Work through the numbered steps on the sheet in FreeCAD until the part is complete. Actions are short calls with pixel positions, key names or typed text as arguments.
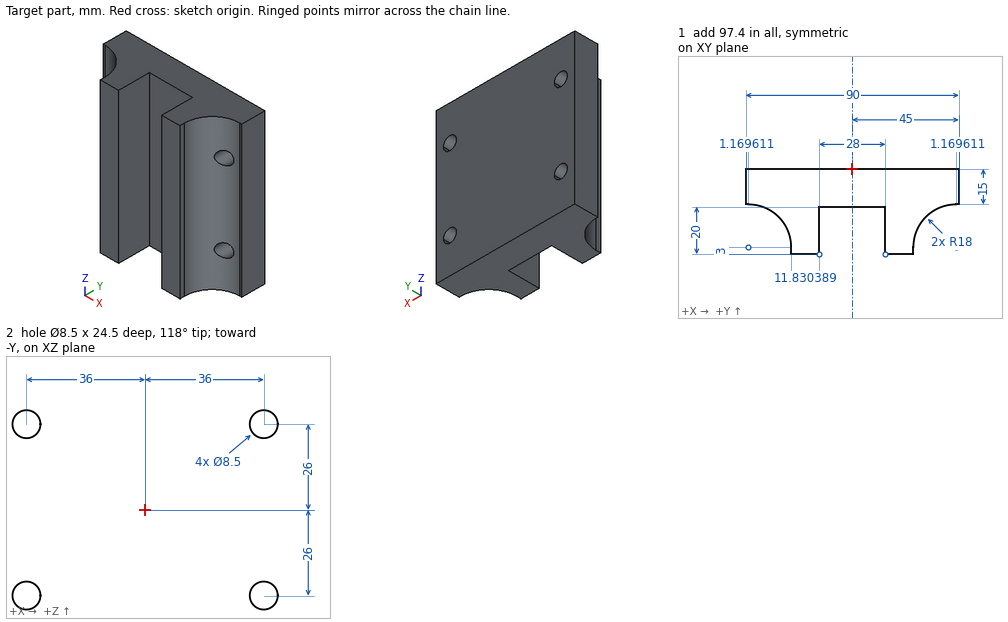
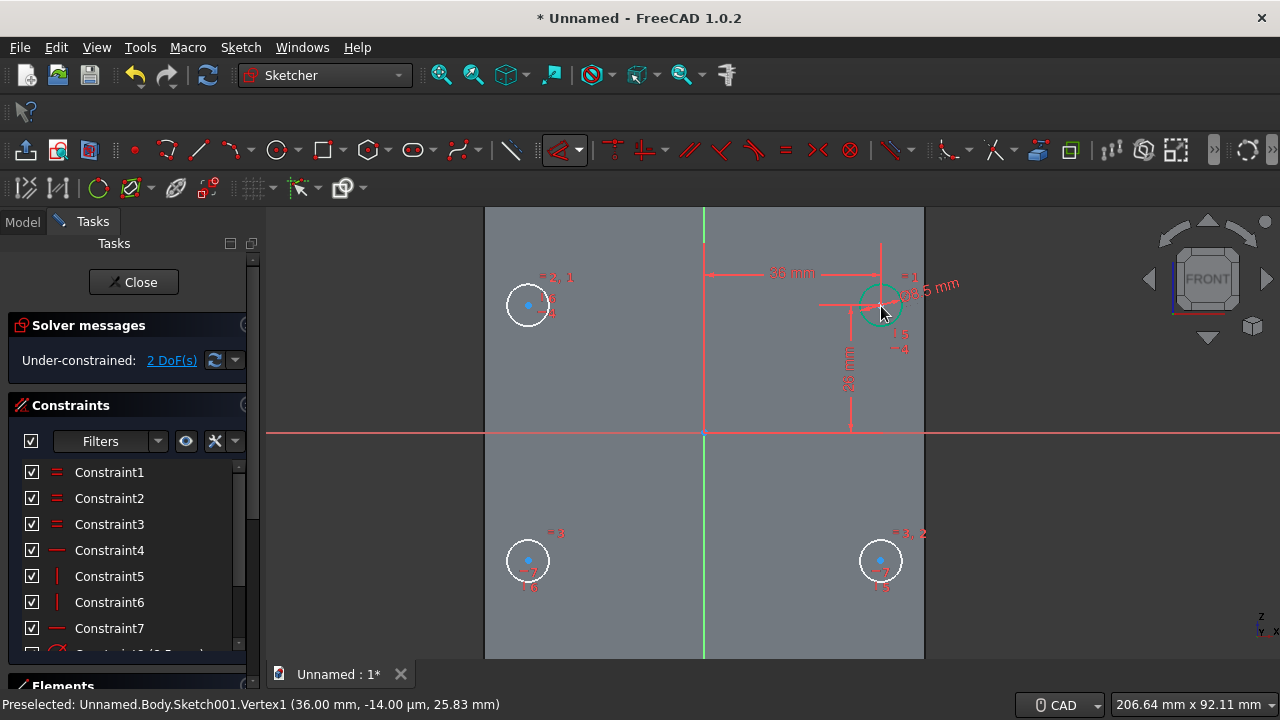
click(528, 305)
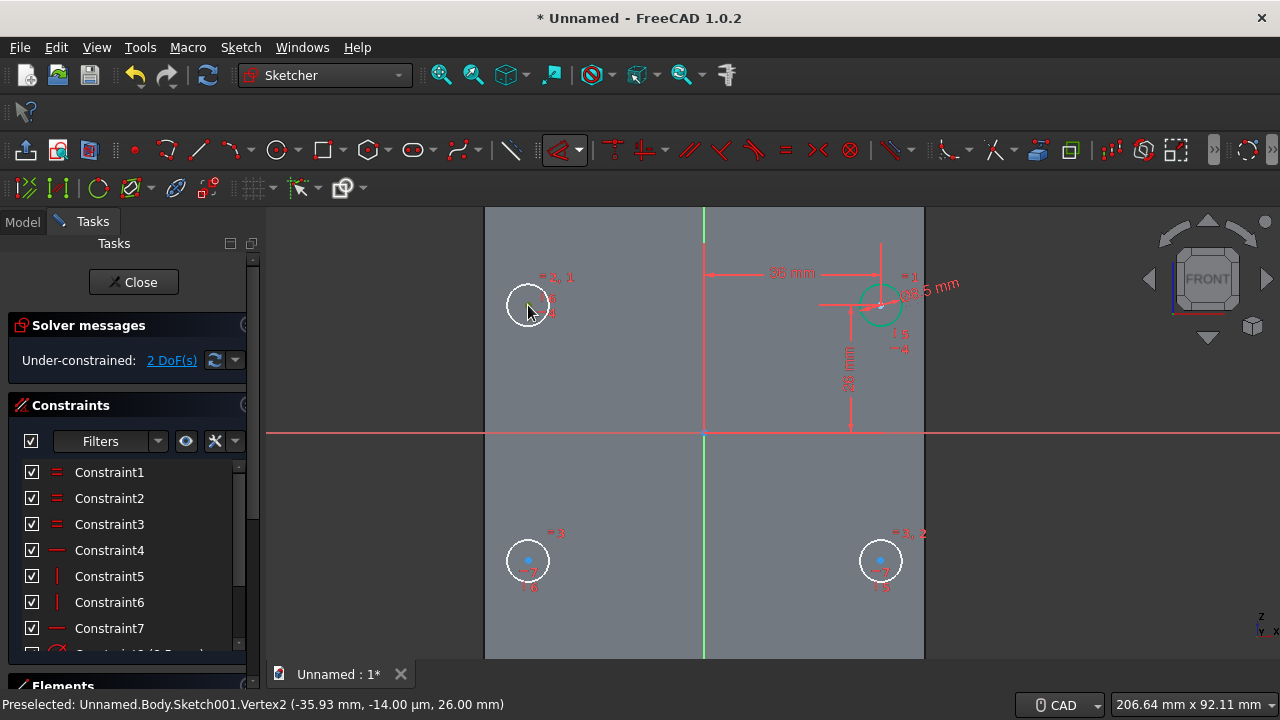
click(582, 150)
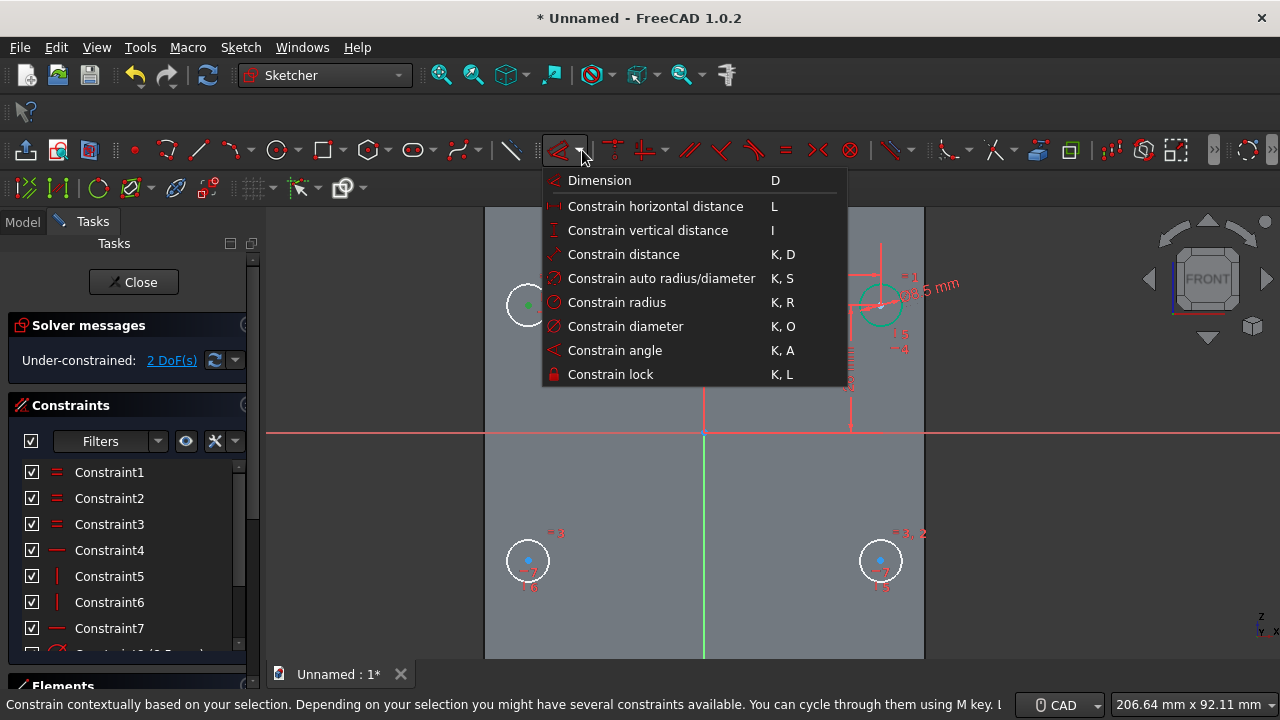
click(695, 206)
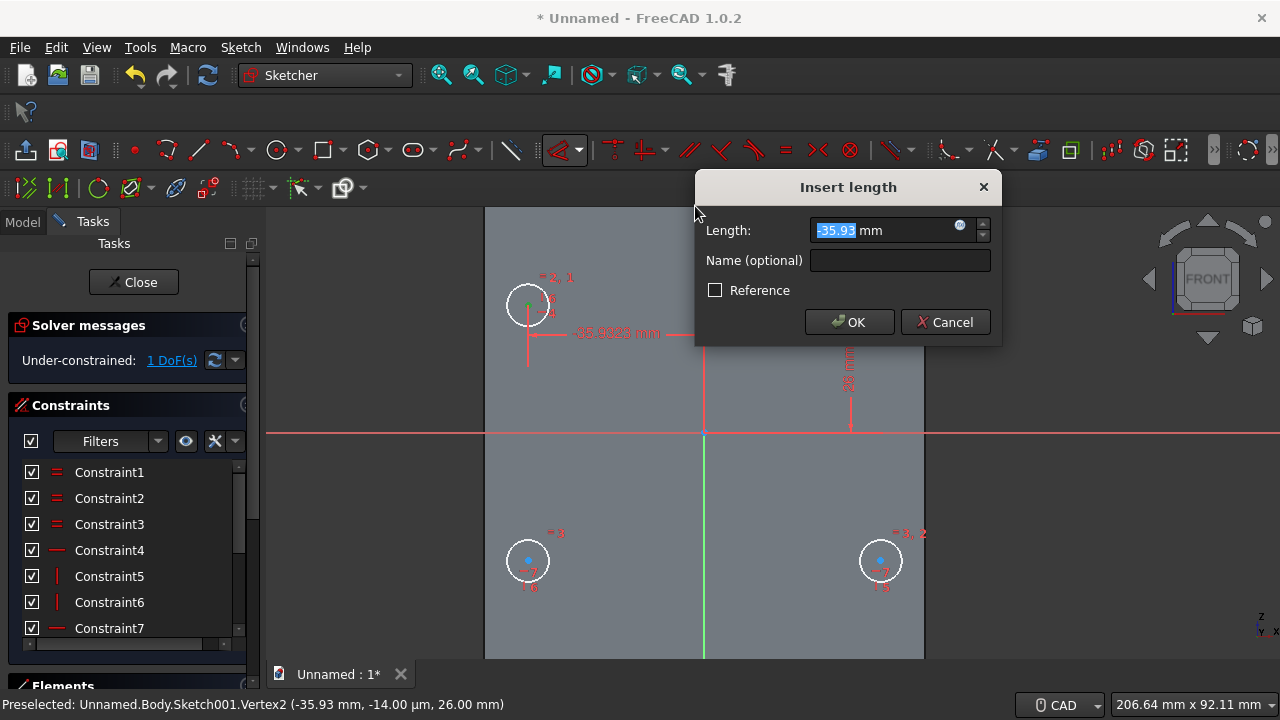
text(-36)
key(Return)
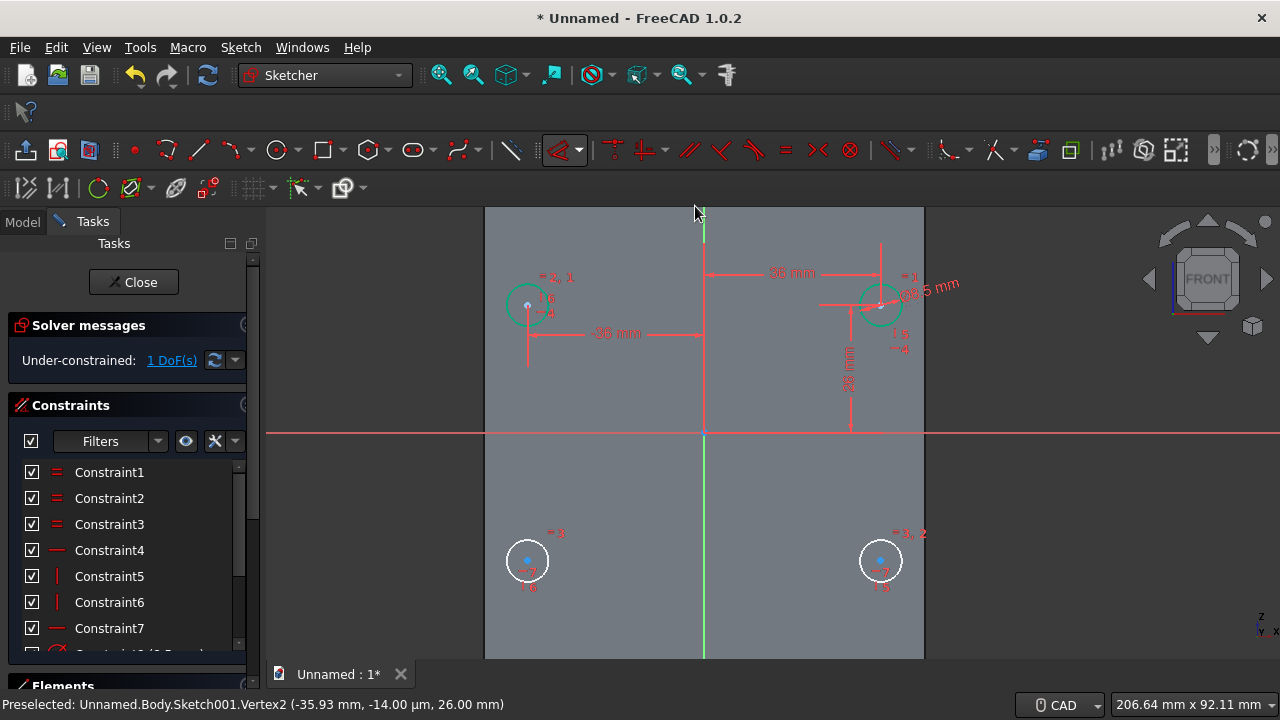
click(881, 561)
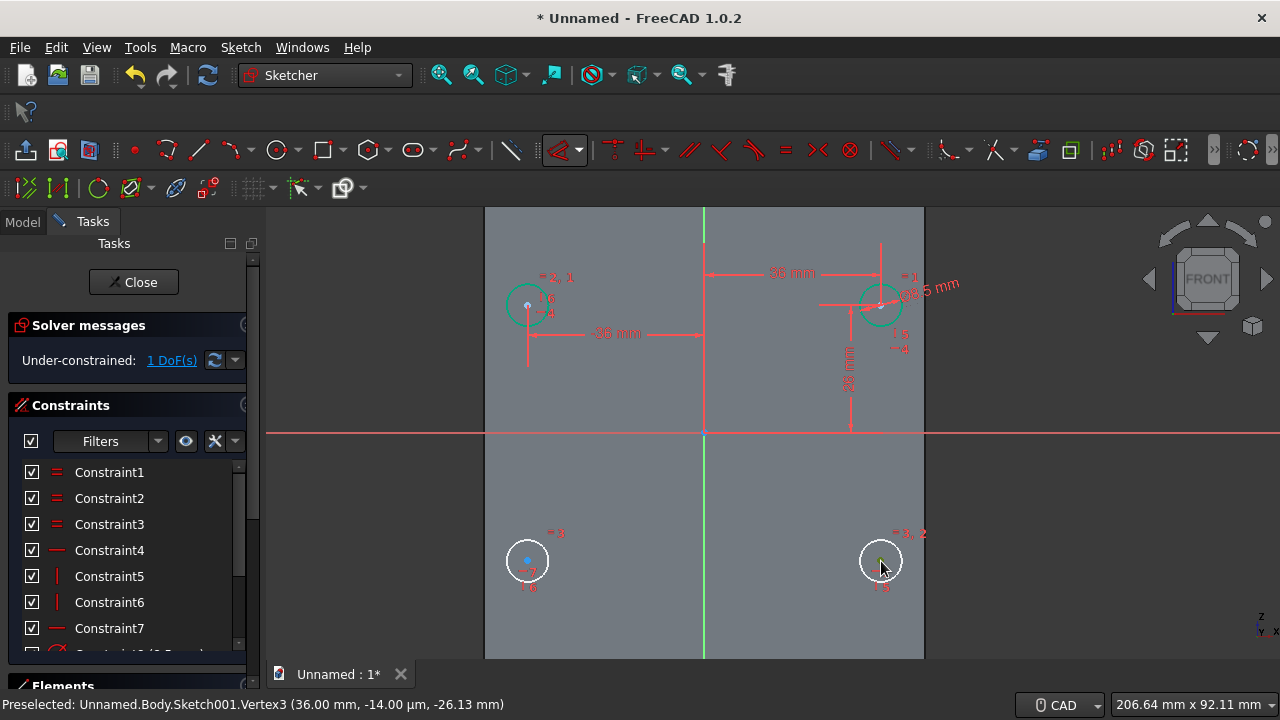
click(582, 150)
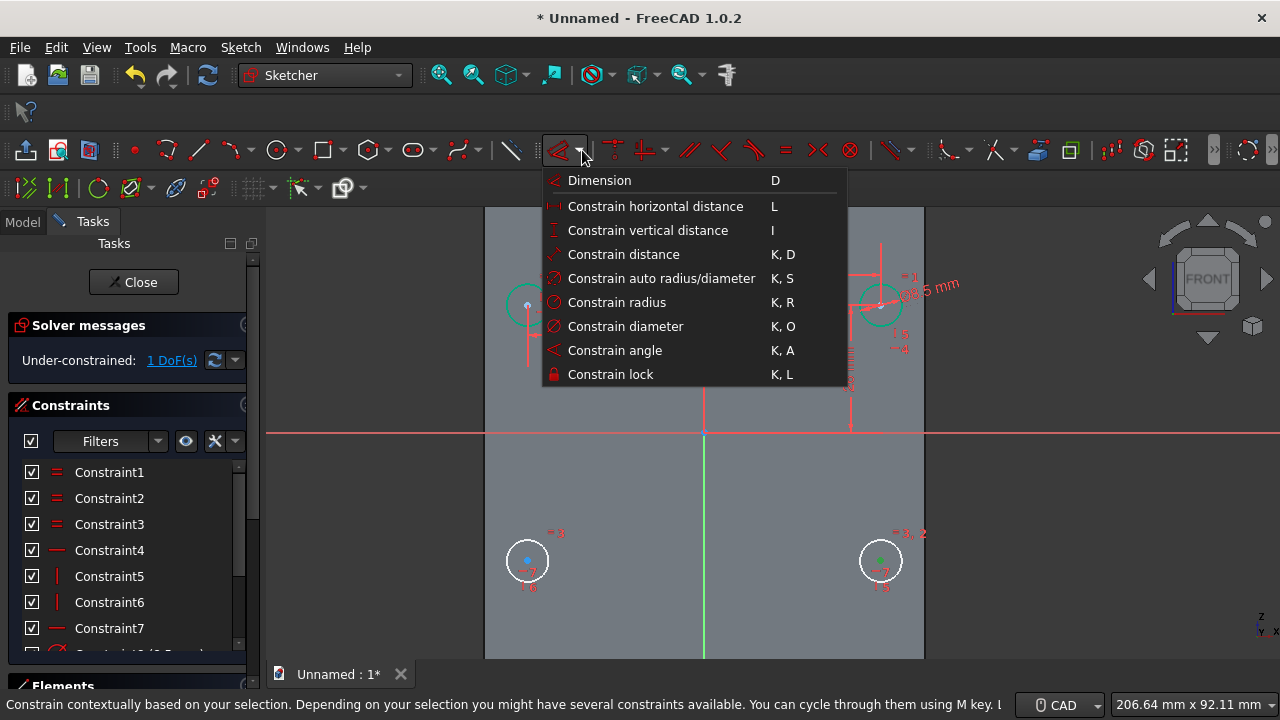
click(695, 230)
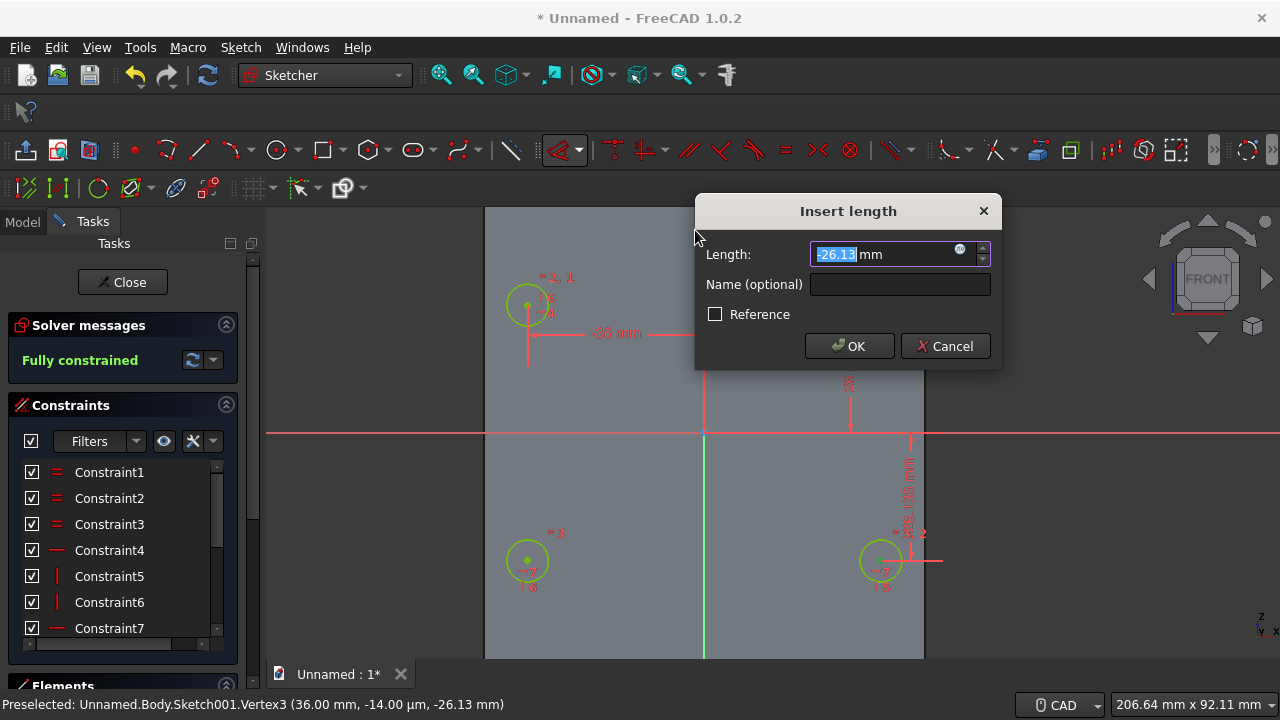
text(-26)
key(Return)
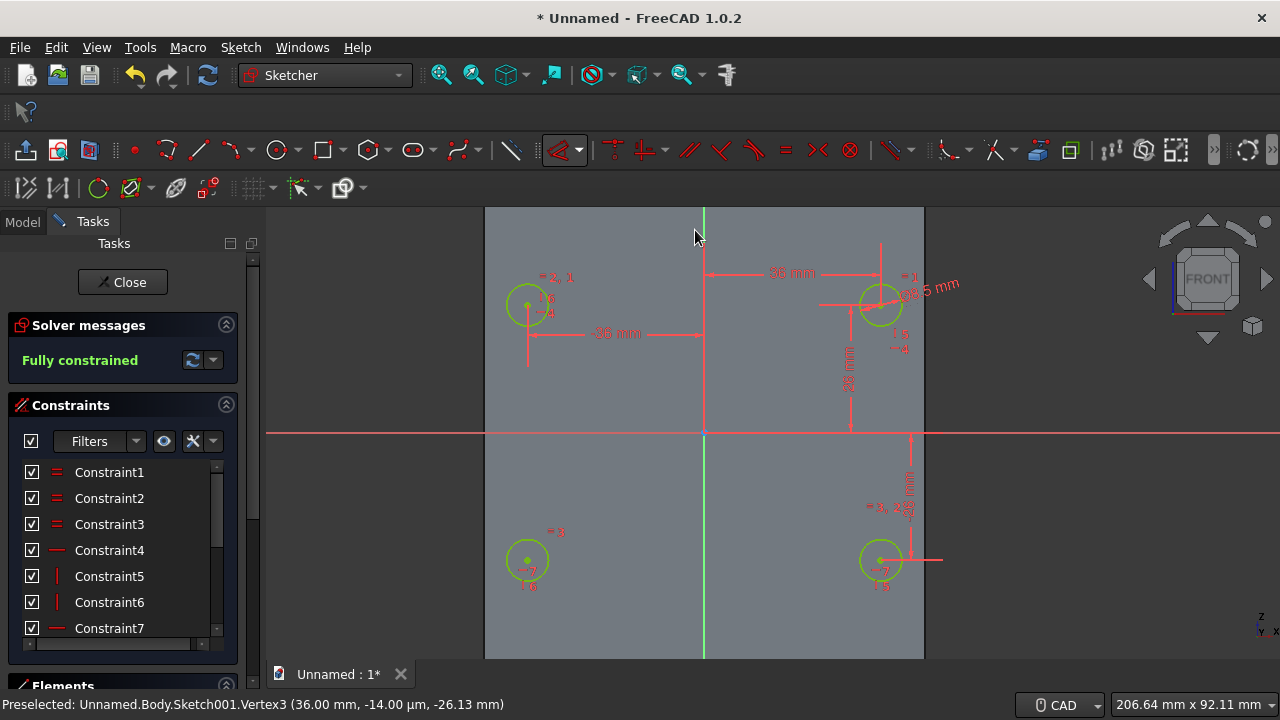
click(123, 282)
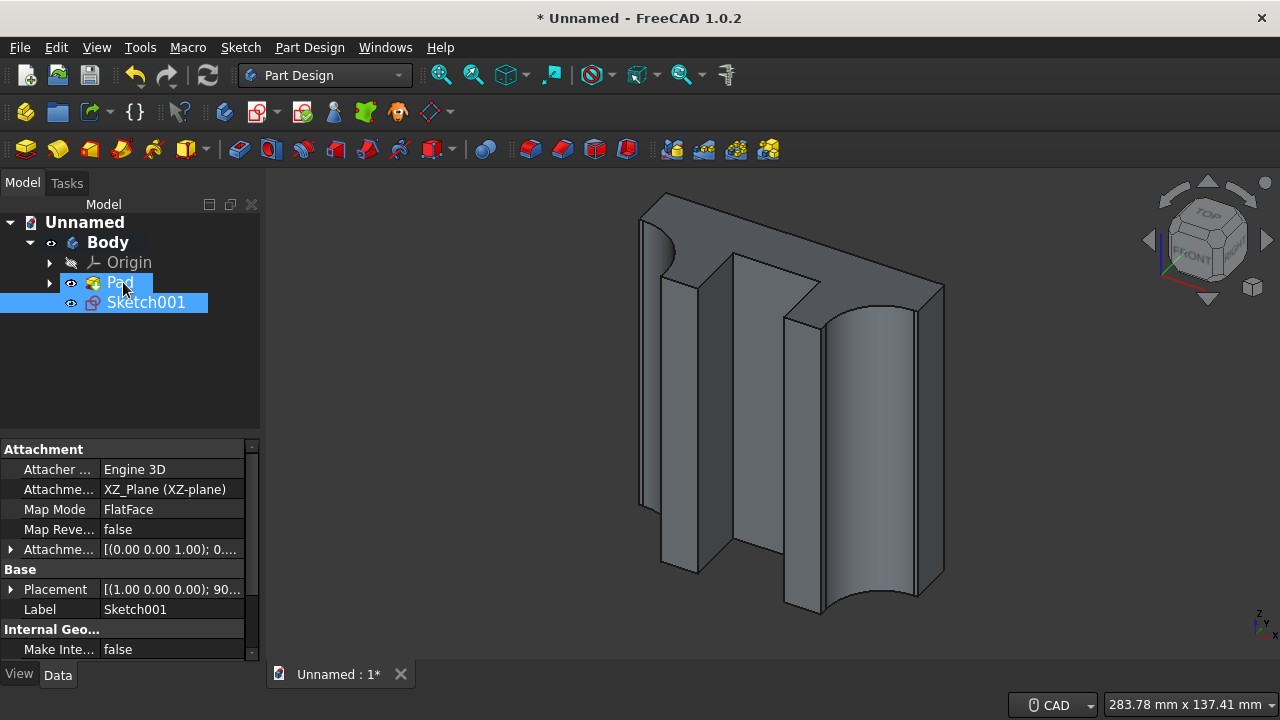
click(272, 150)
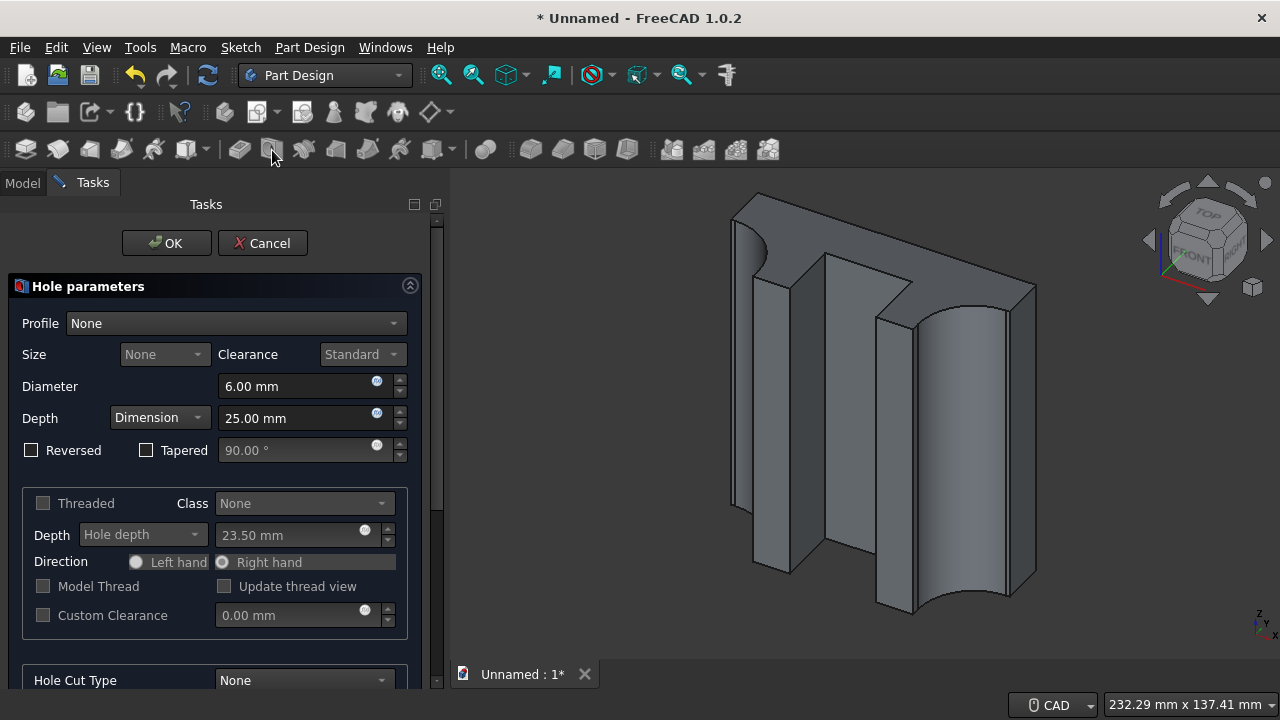
triple_click(305, 386)